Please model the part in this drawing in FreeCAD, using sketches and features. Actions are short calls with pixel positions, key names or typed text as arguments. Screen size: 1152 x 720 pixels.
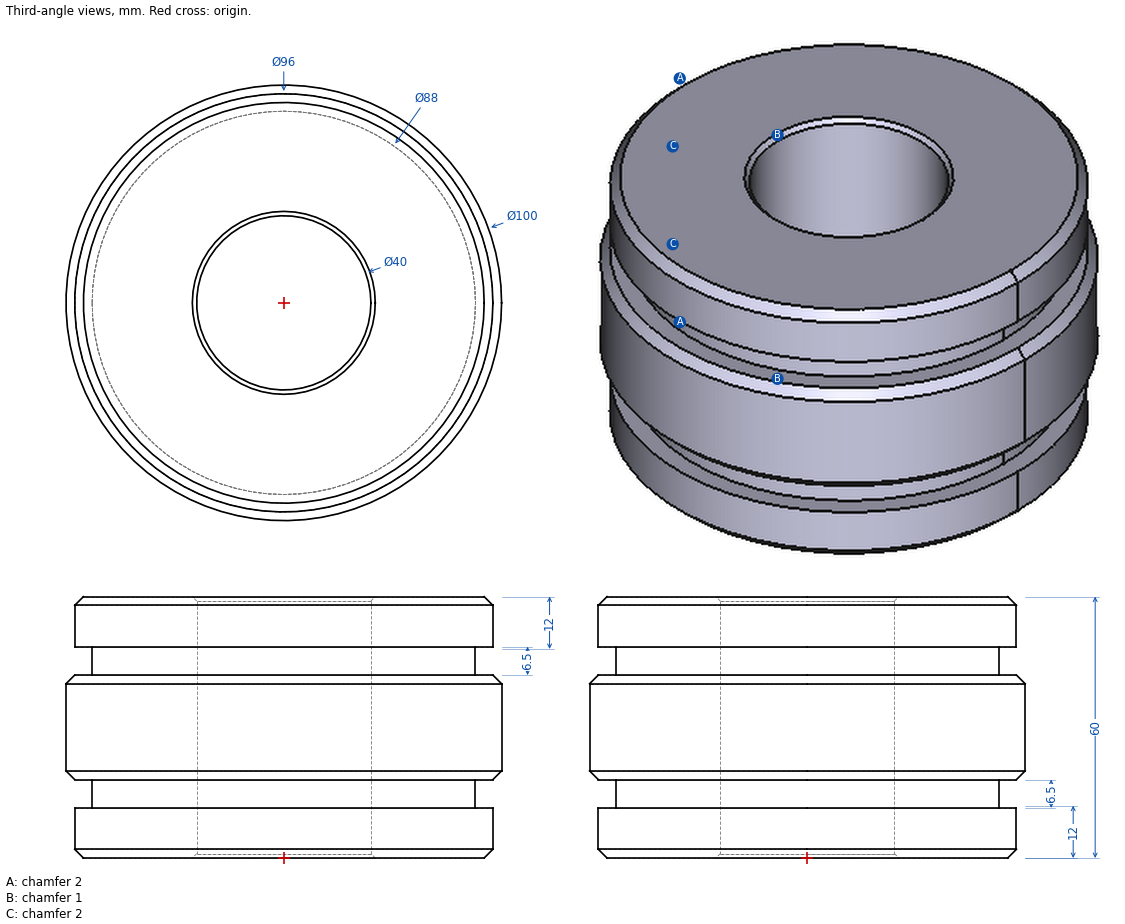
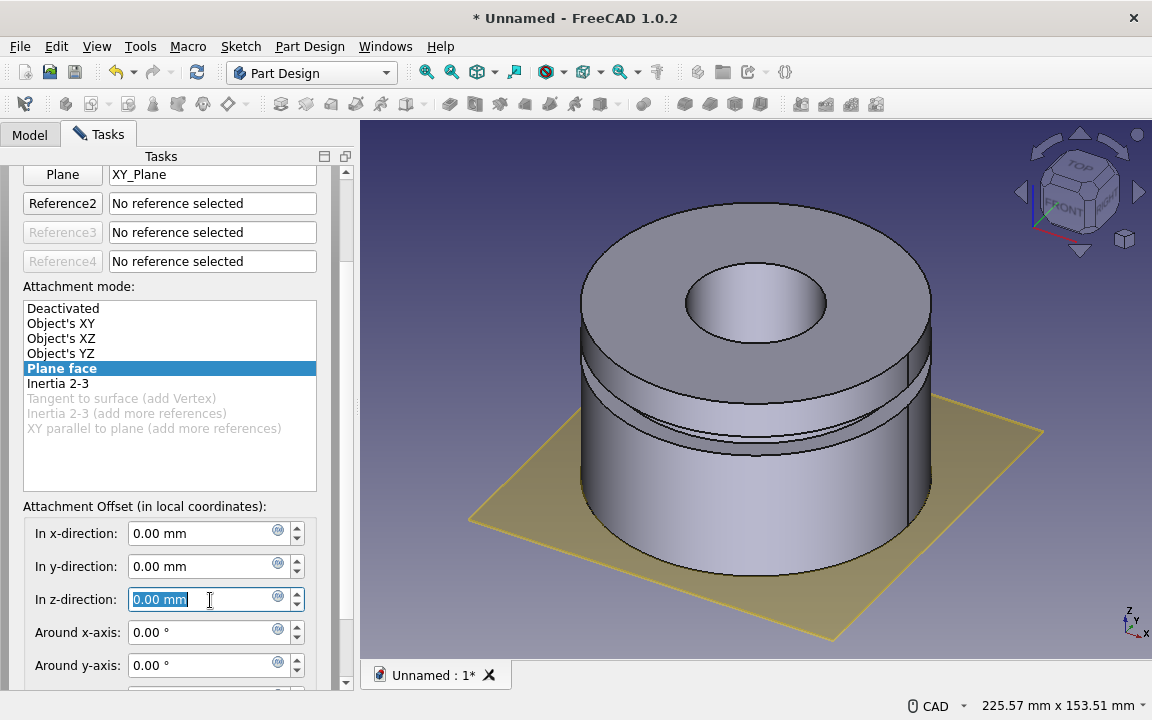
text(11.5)
key(Tab)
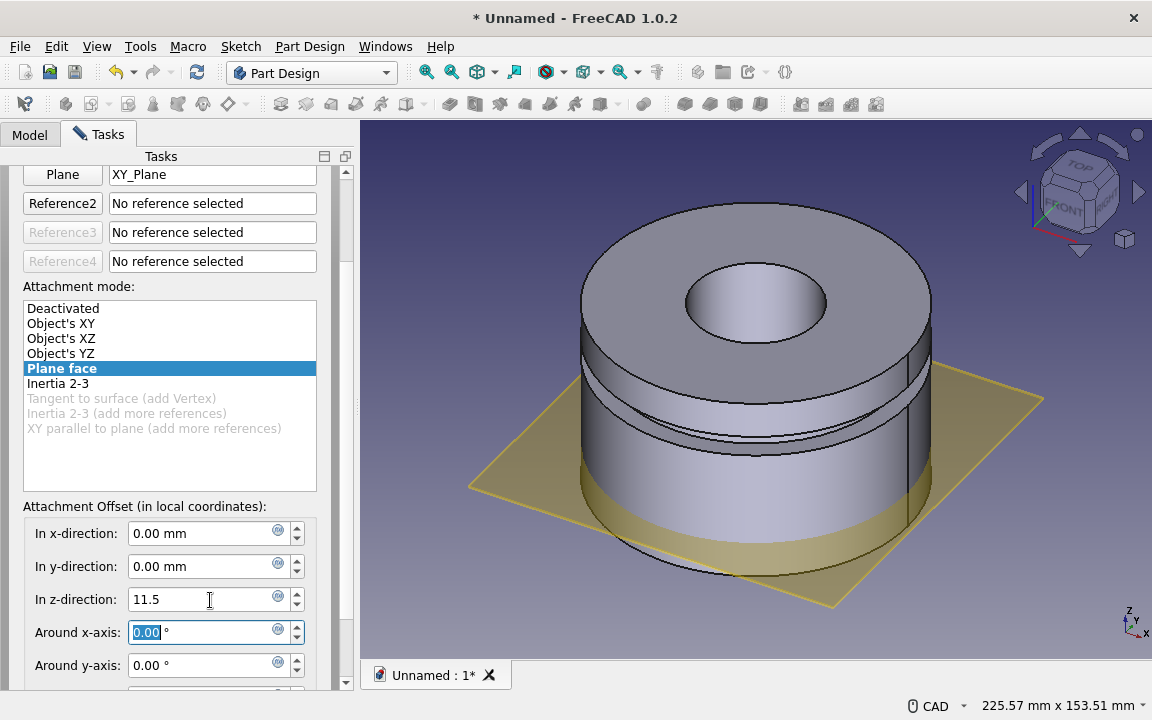
scroll(346, 428, up, 3)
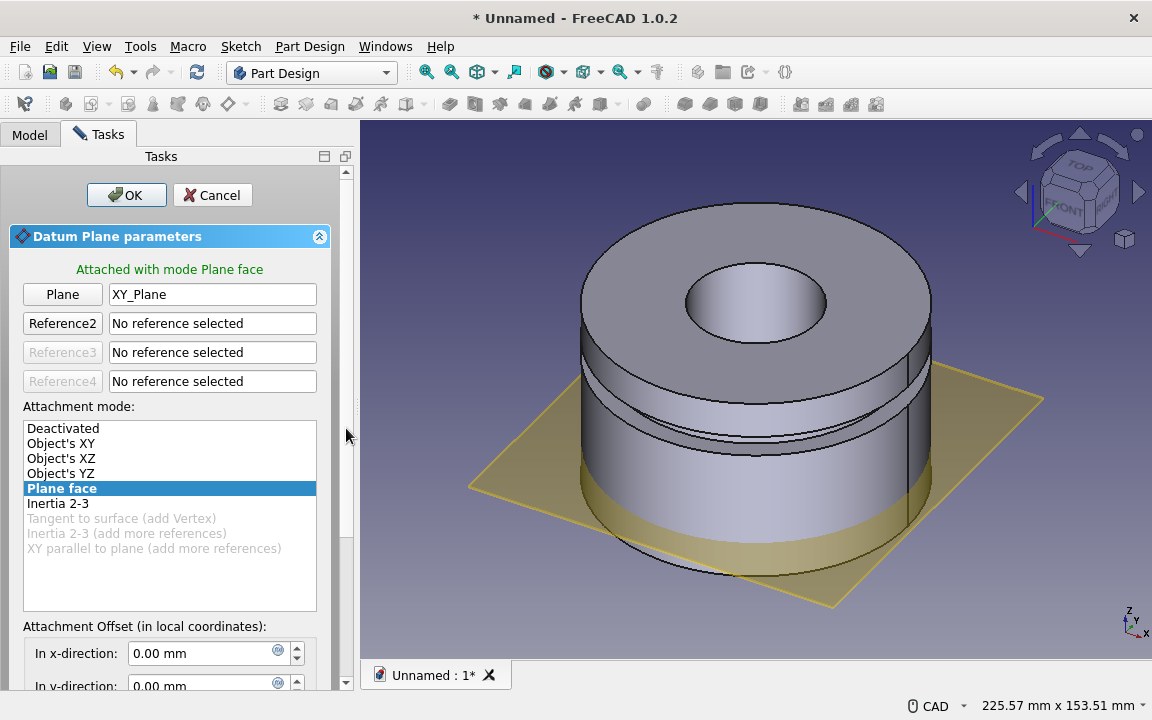
click(127, 195)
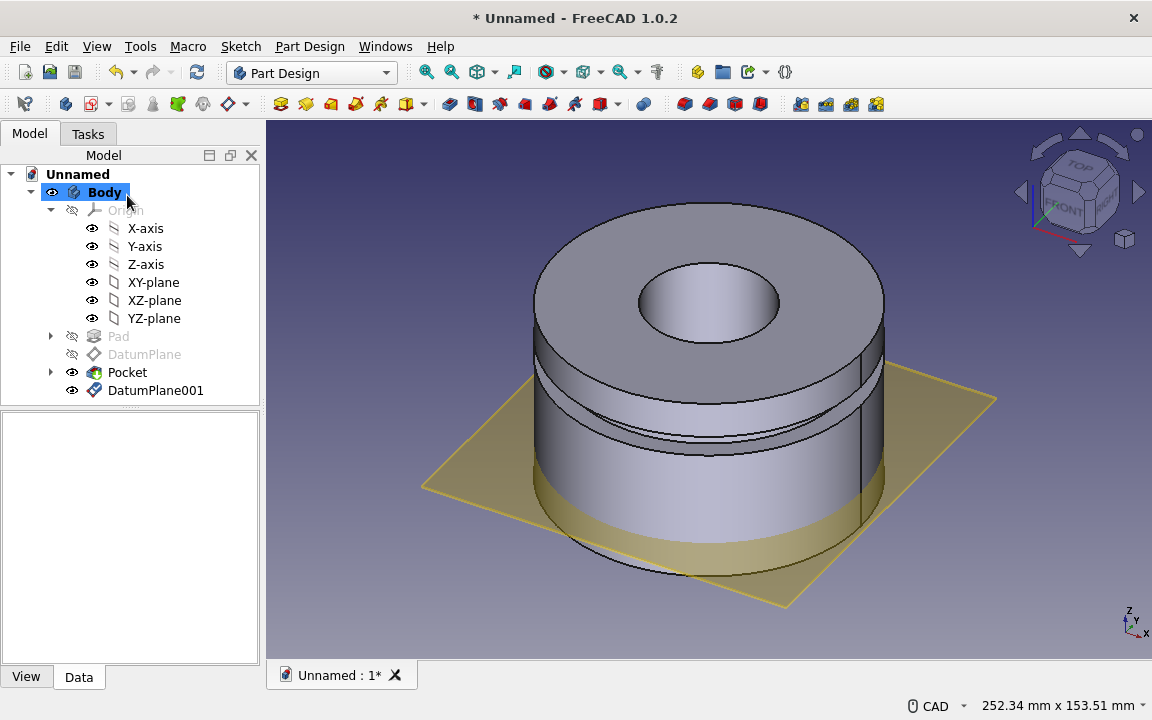
click(117, 390)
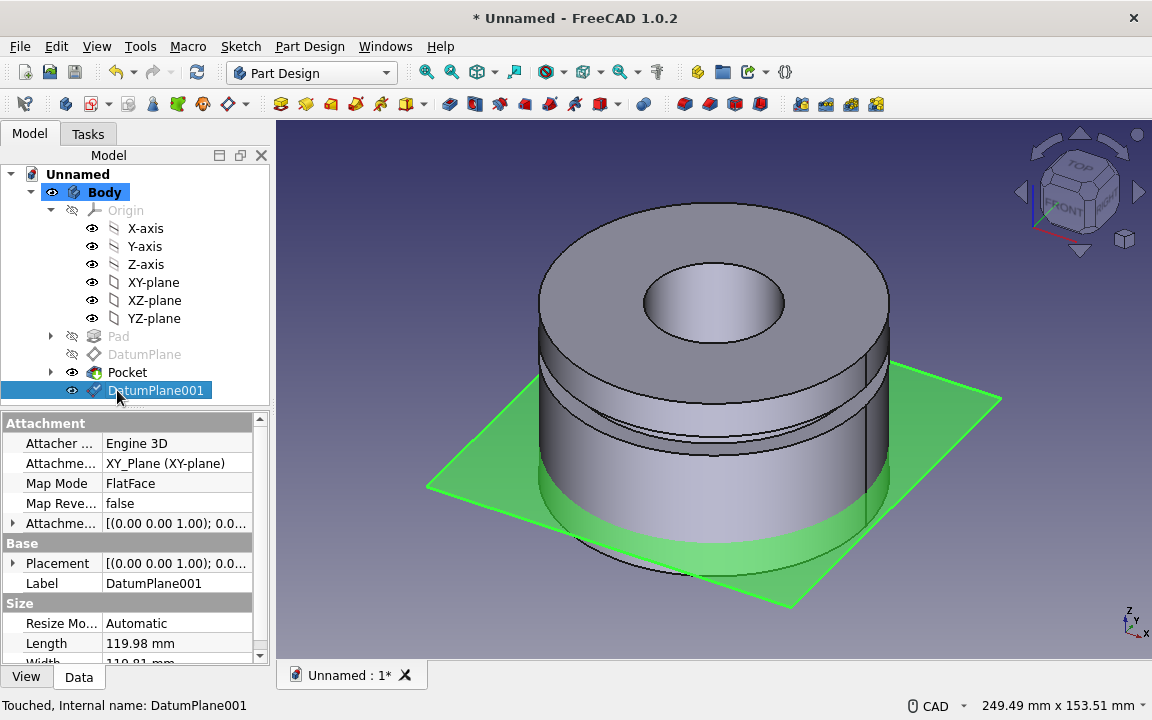
click(90, 104)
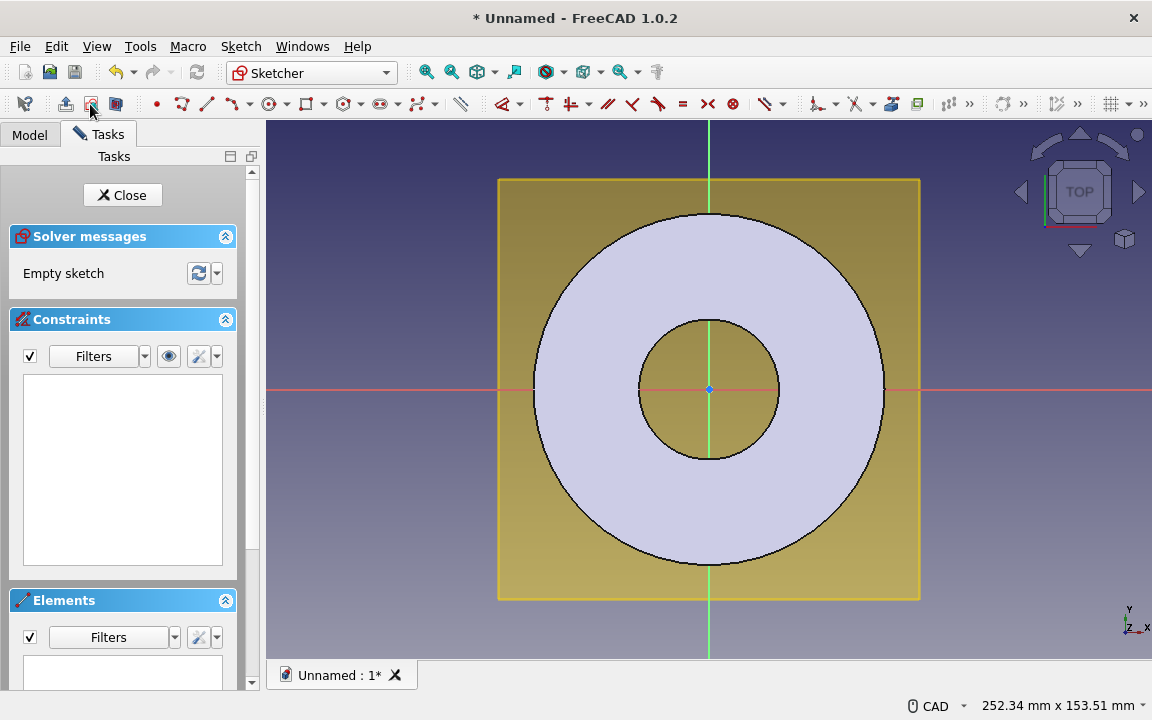
click(116, 104)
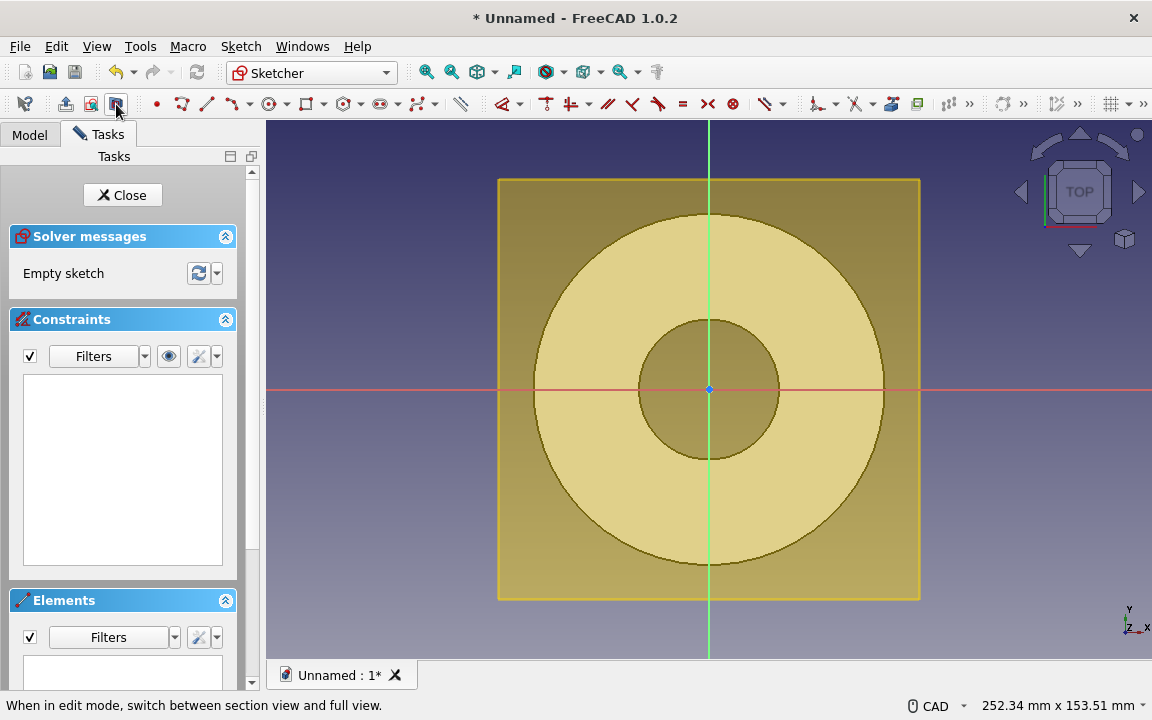
click(268, 104)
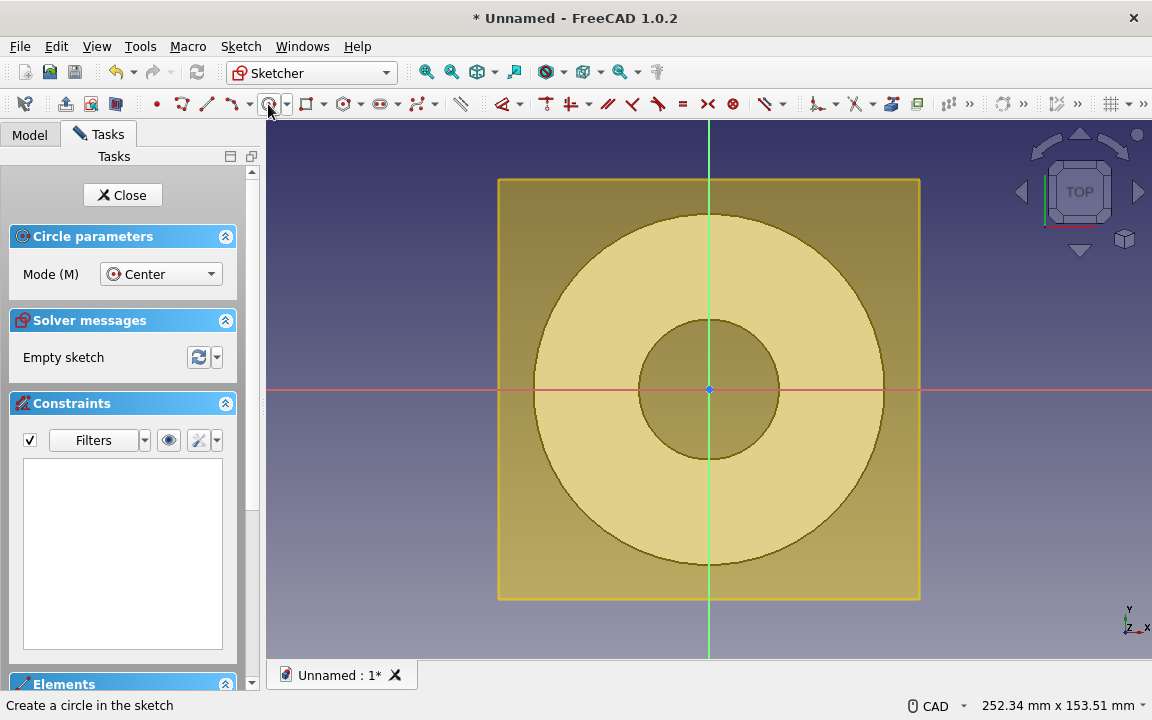
click(709, 390)
click(833, 265)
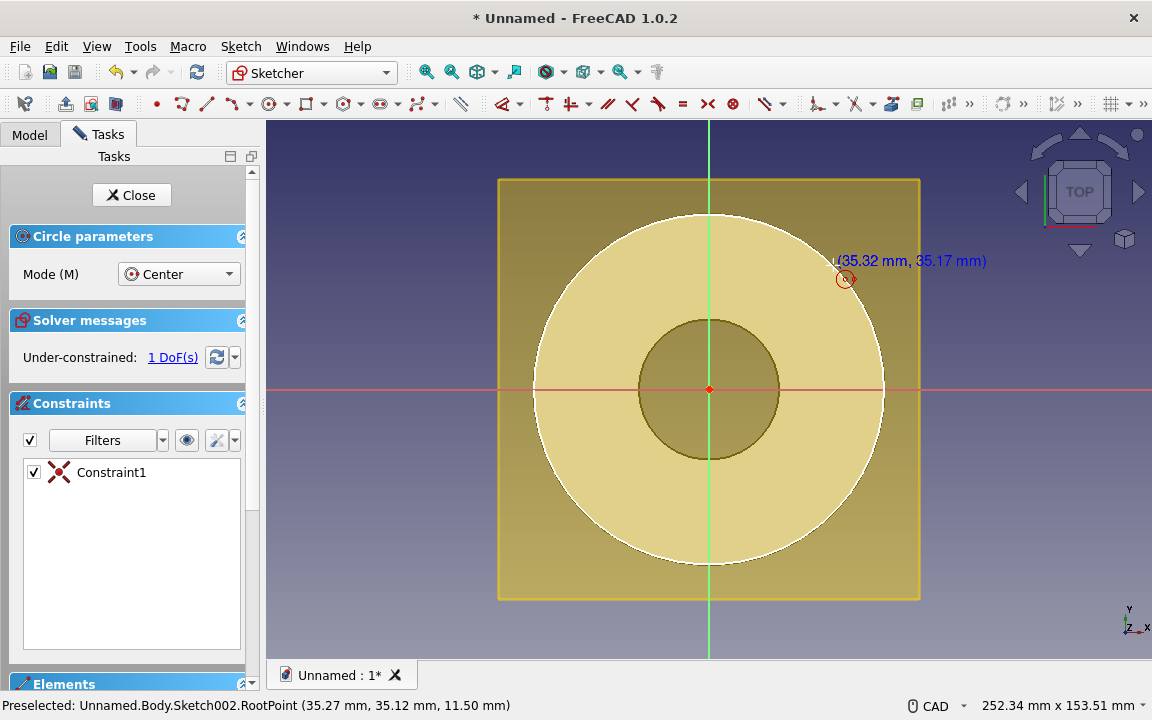
click(709, 390)
click(818, 280)
key(Escape)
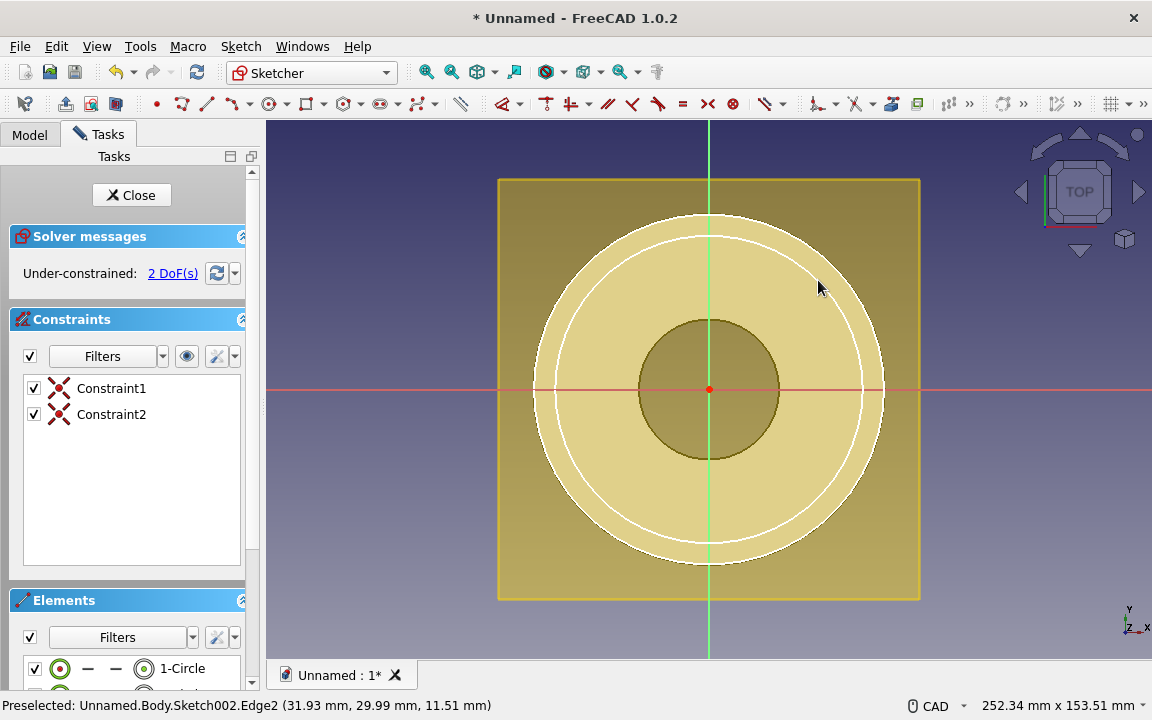
click(502, 104)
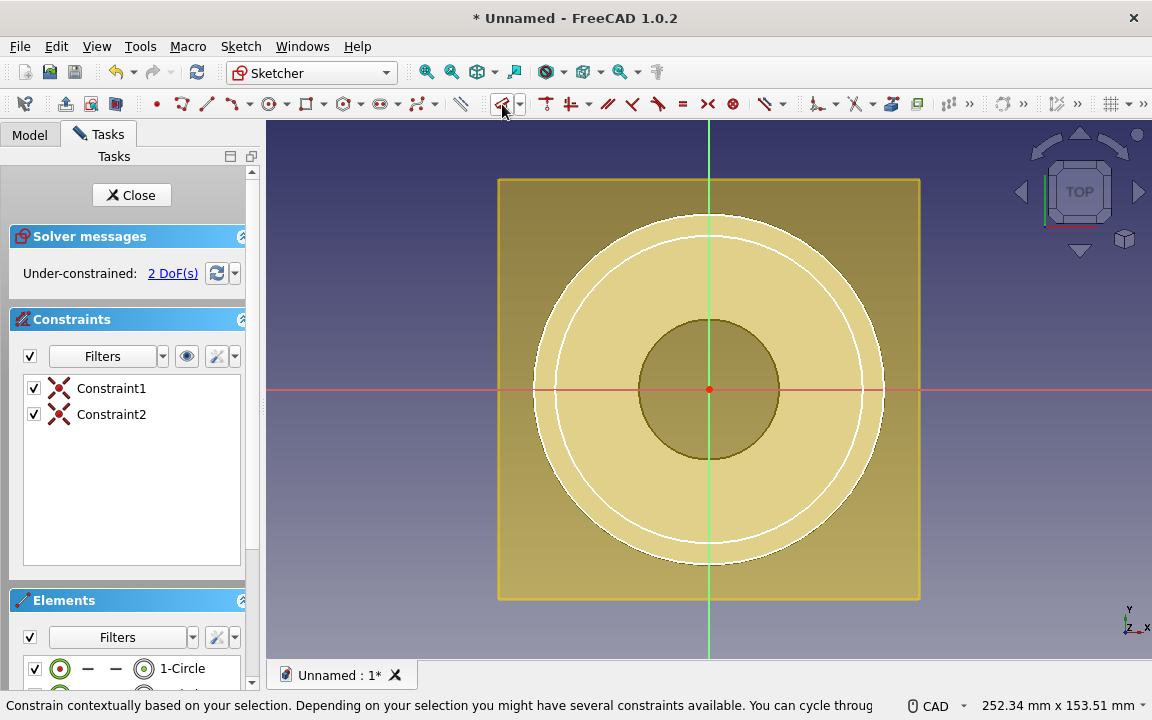
click(832, 265)
click(854, 242)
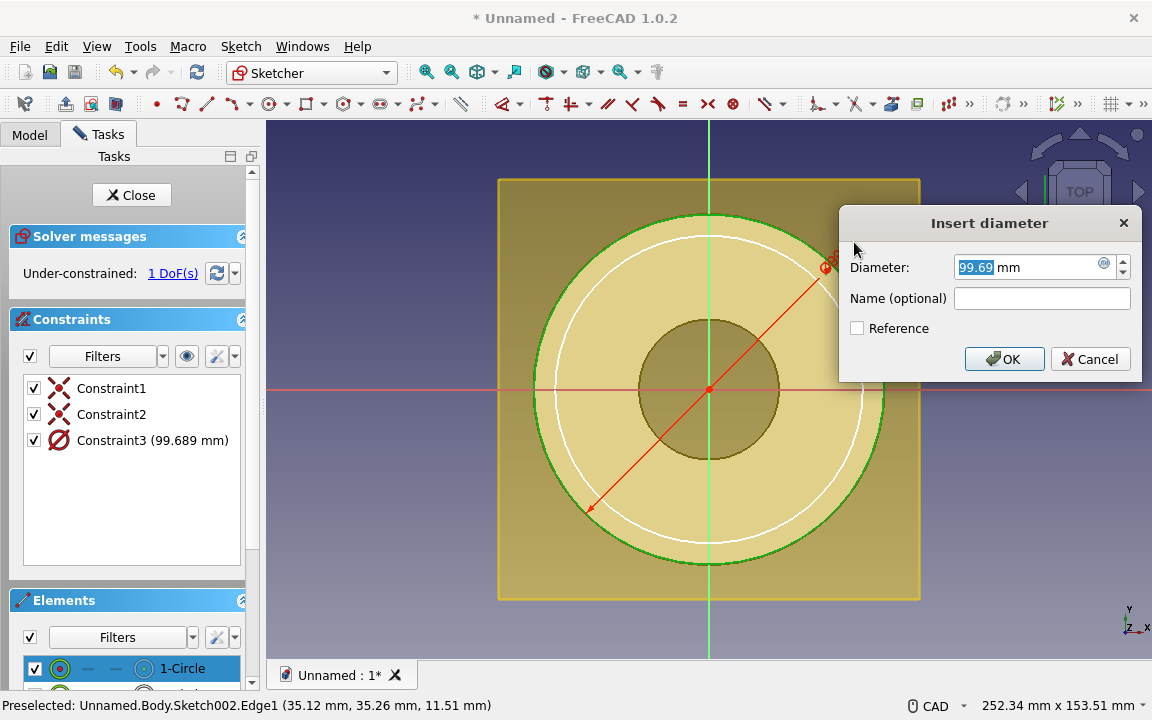
text(100)
key(Return)